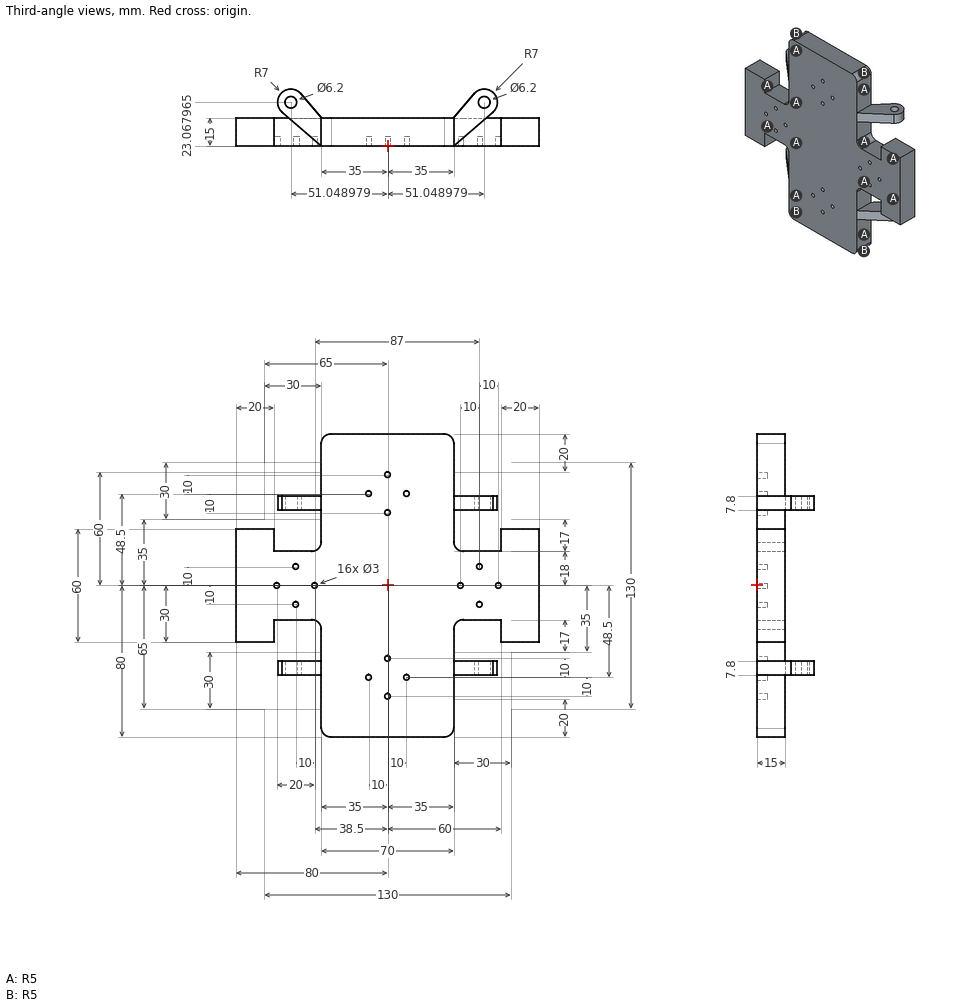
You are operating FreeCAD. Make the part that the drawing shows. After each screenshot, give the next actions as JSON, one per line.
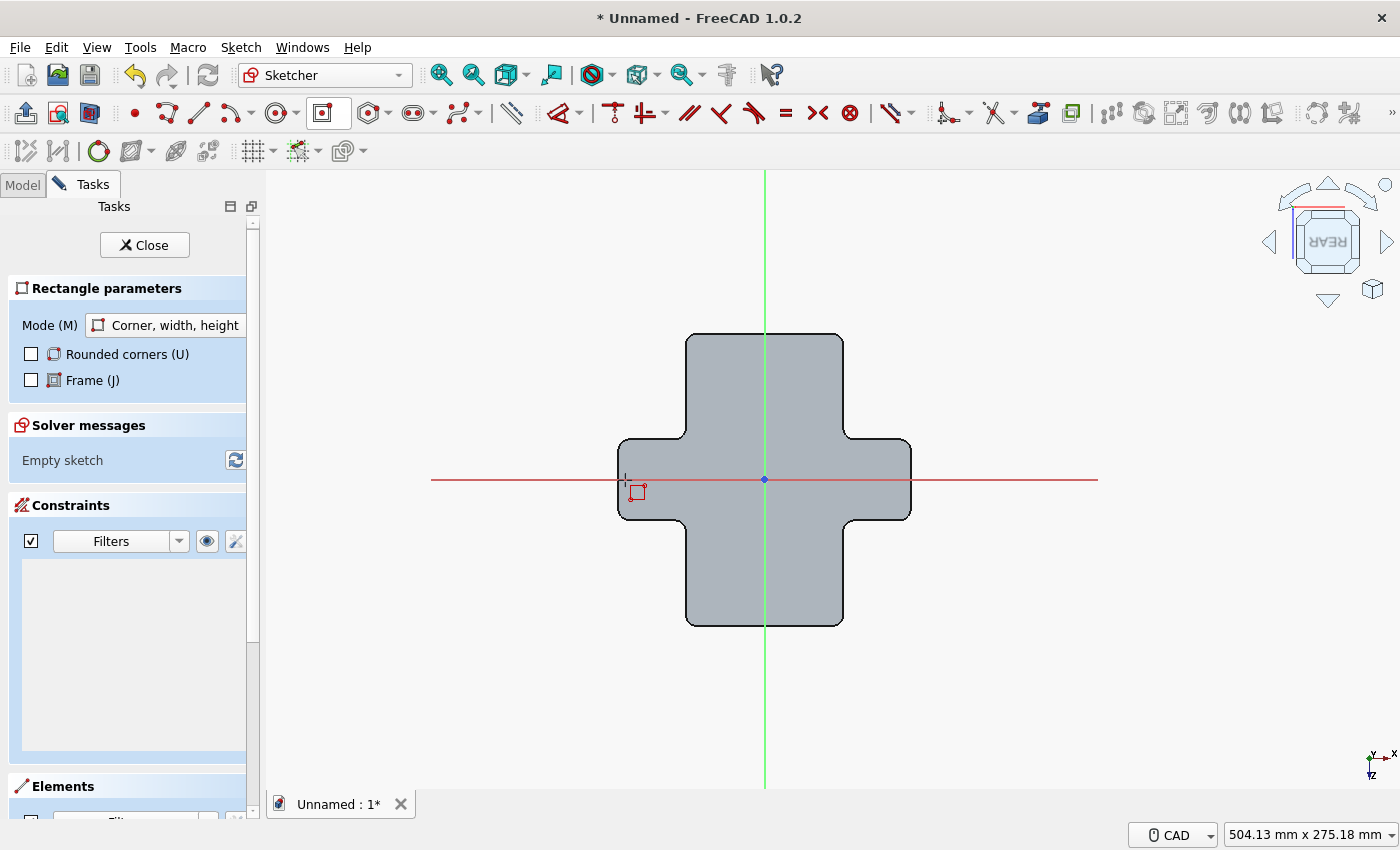
{"action": "left_click", "coordinate": [686, 300]}
{"action": "mouse_move", "coordinate": [843, 345]}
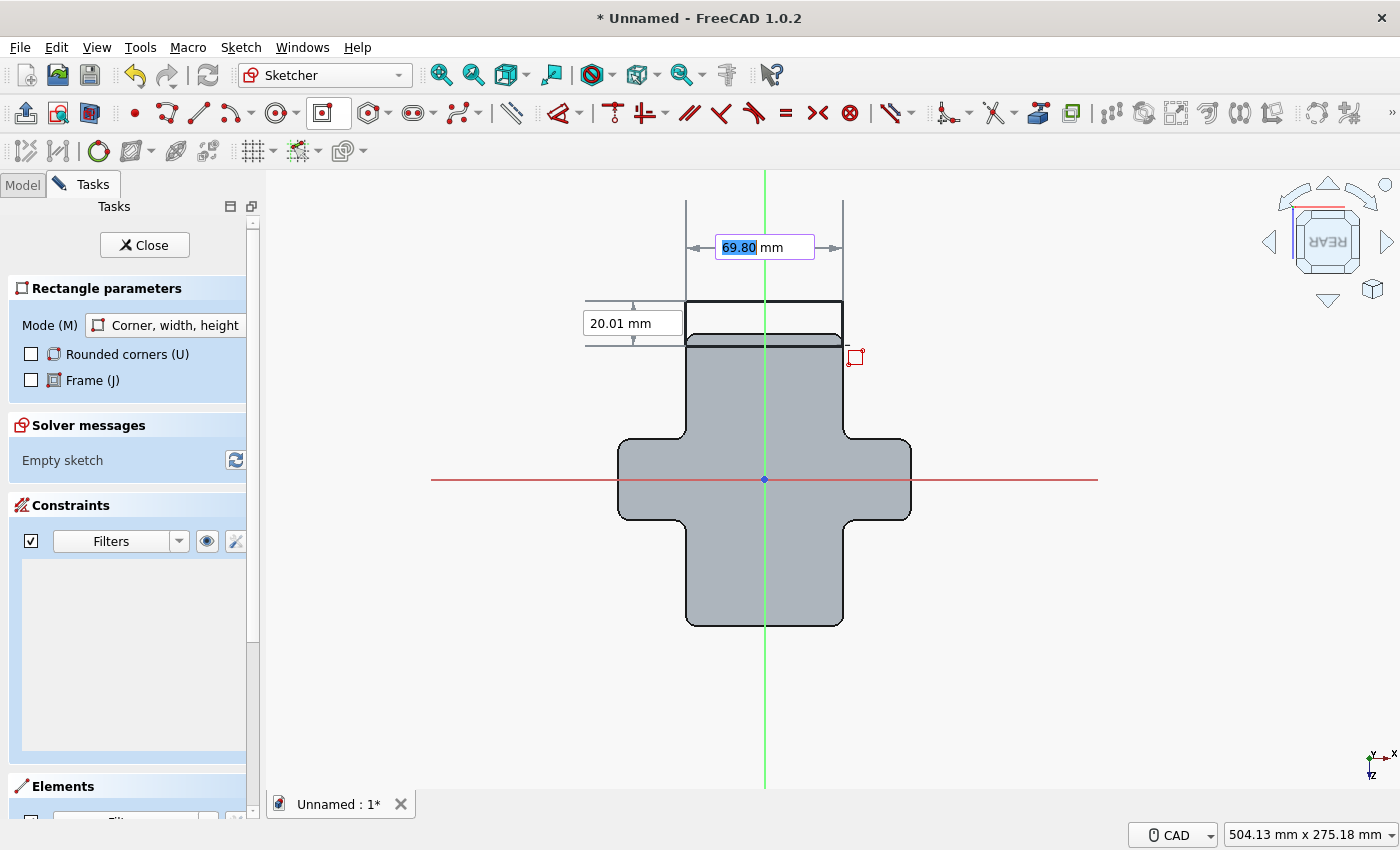
{"action": "type", "text": "70"}
{"action": "key", "text": "Tab"}
{"action": "type", "text": "20"}
{"action": "key", "text": "Return"}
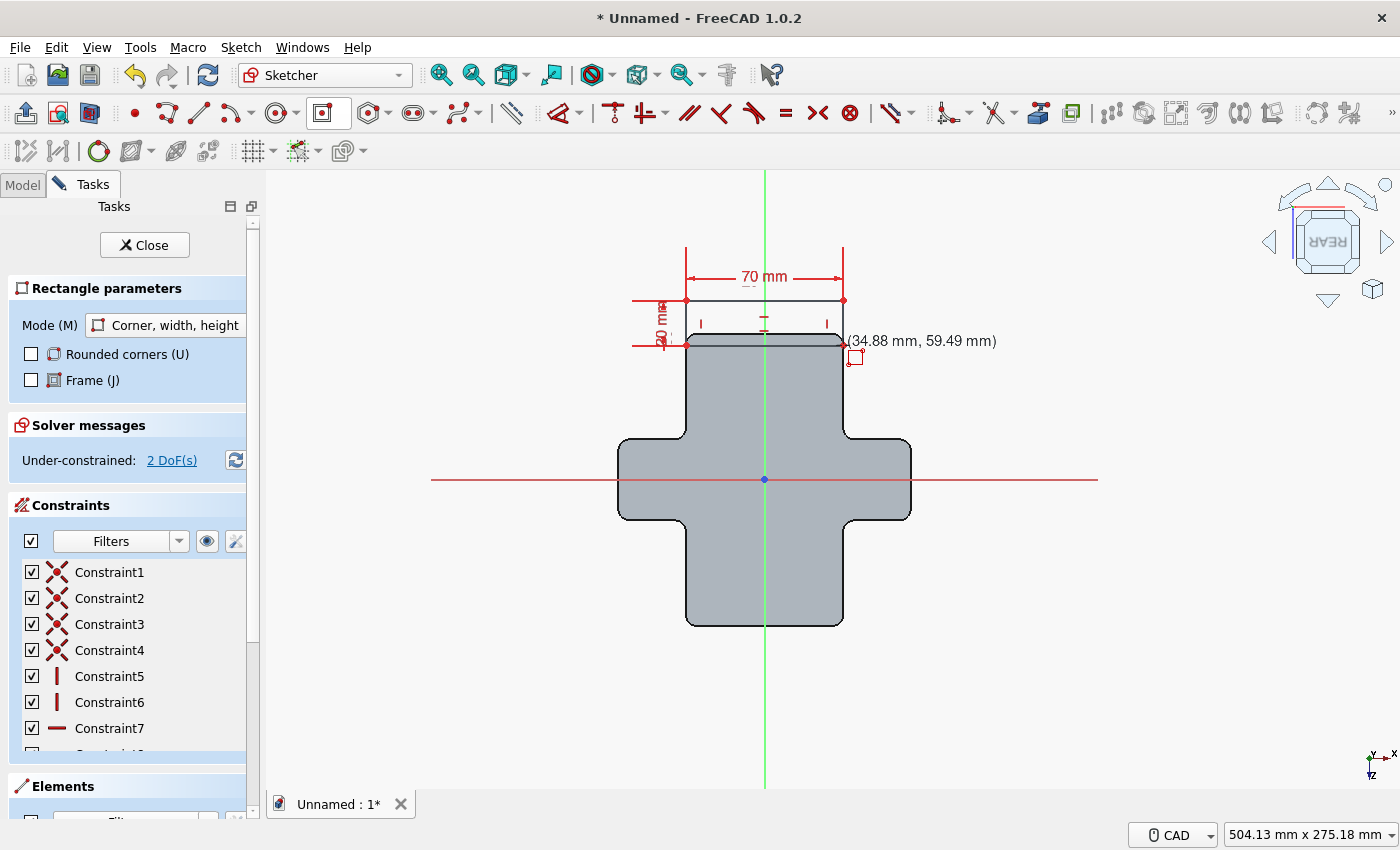
{"action": "left_click", "coordinate": [686, 615]}
{"action": "mouse_move", "coordinate": [843, 660]}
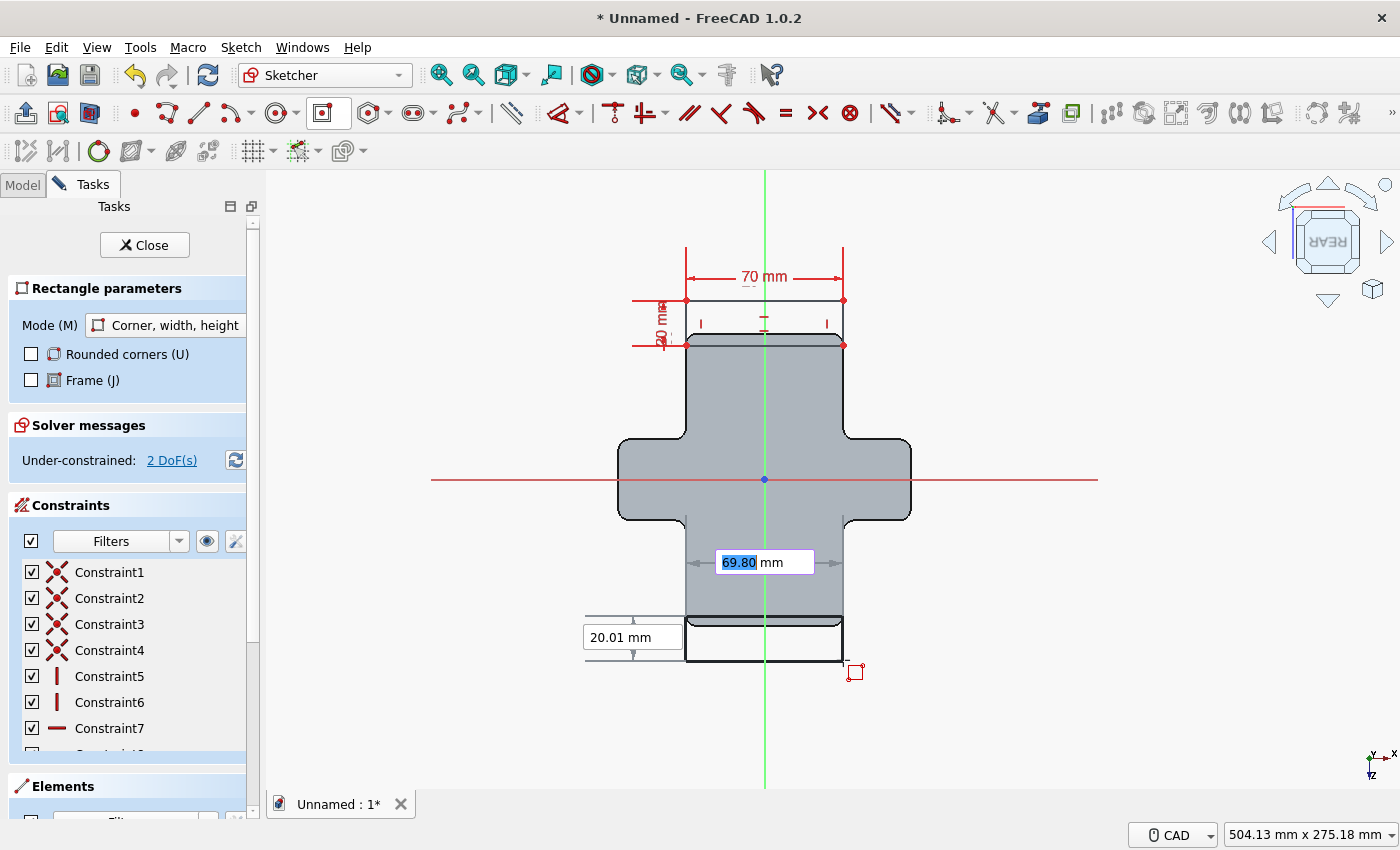
{"action": "type", "text": "70"}
{"action": "key", "text": "Tab"}
{"action": "type", "text": "20"}
{"action": "key", "text": "Return"}
{"action": "key", "text": "Escape"}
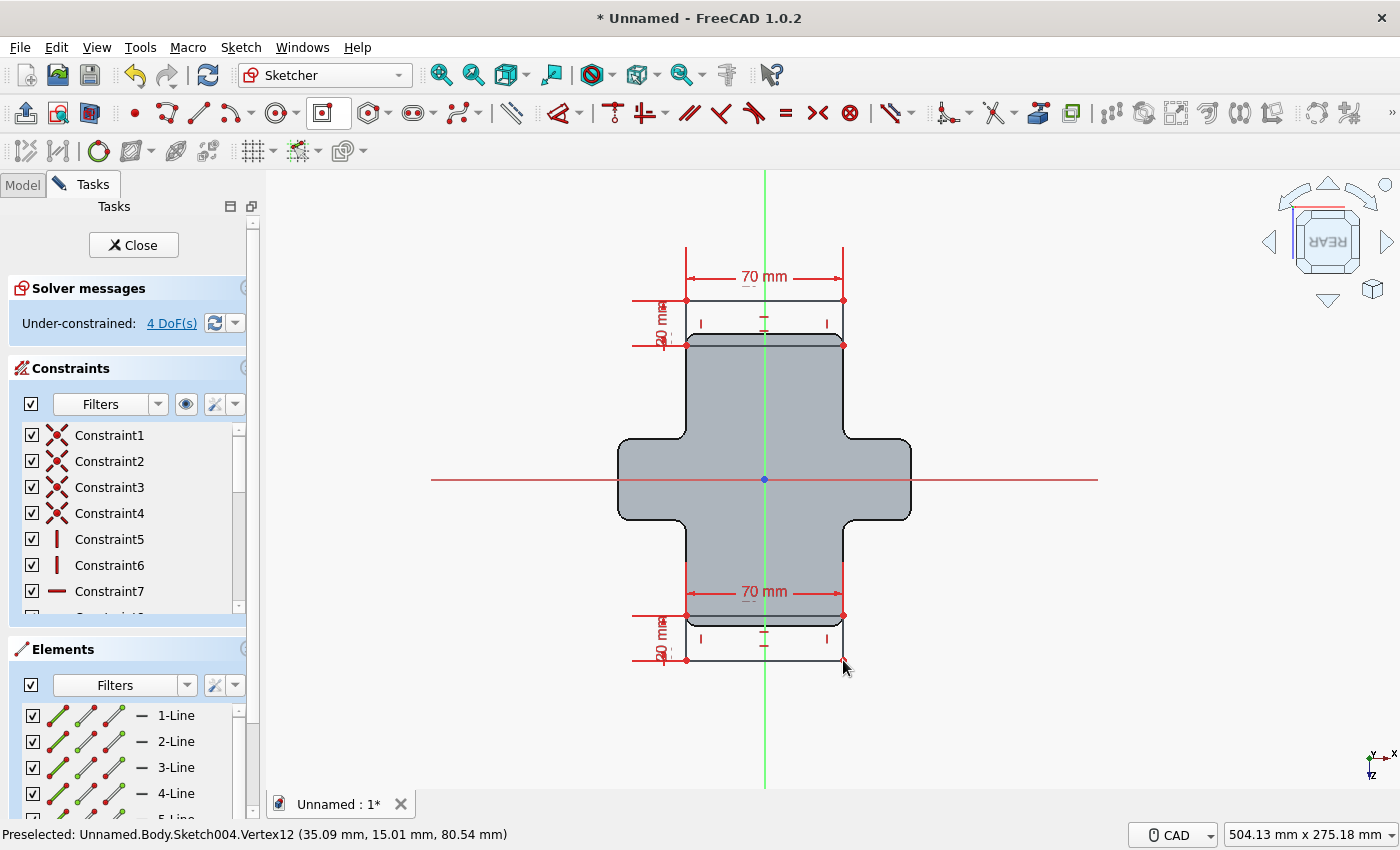
{"action": "key", "text": "d"}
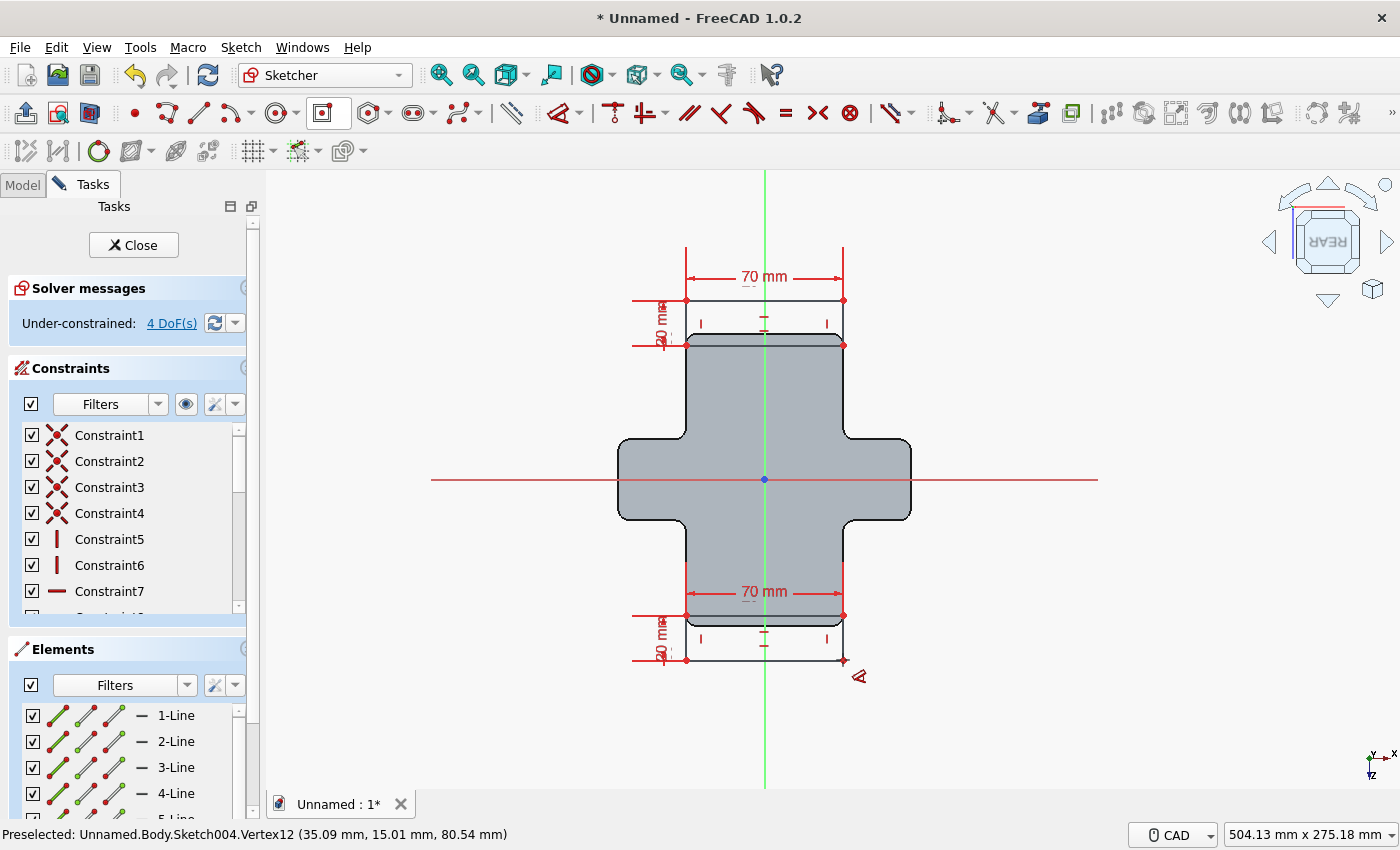
{"action": "left_click", "coordinate": [686, 301]}
{"action": "left_click", "coordinate": [725, 267]}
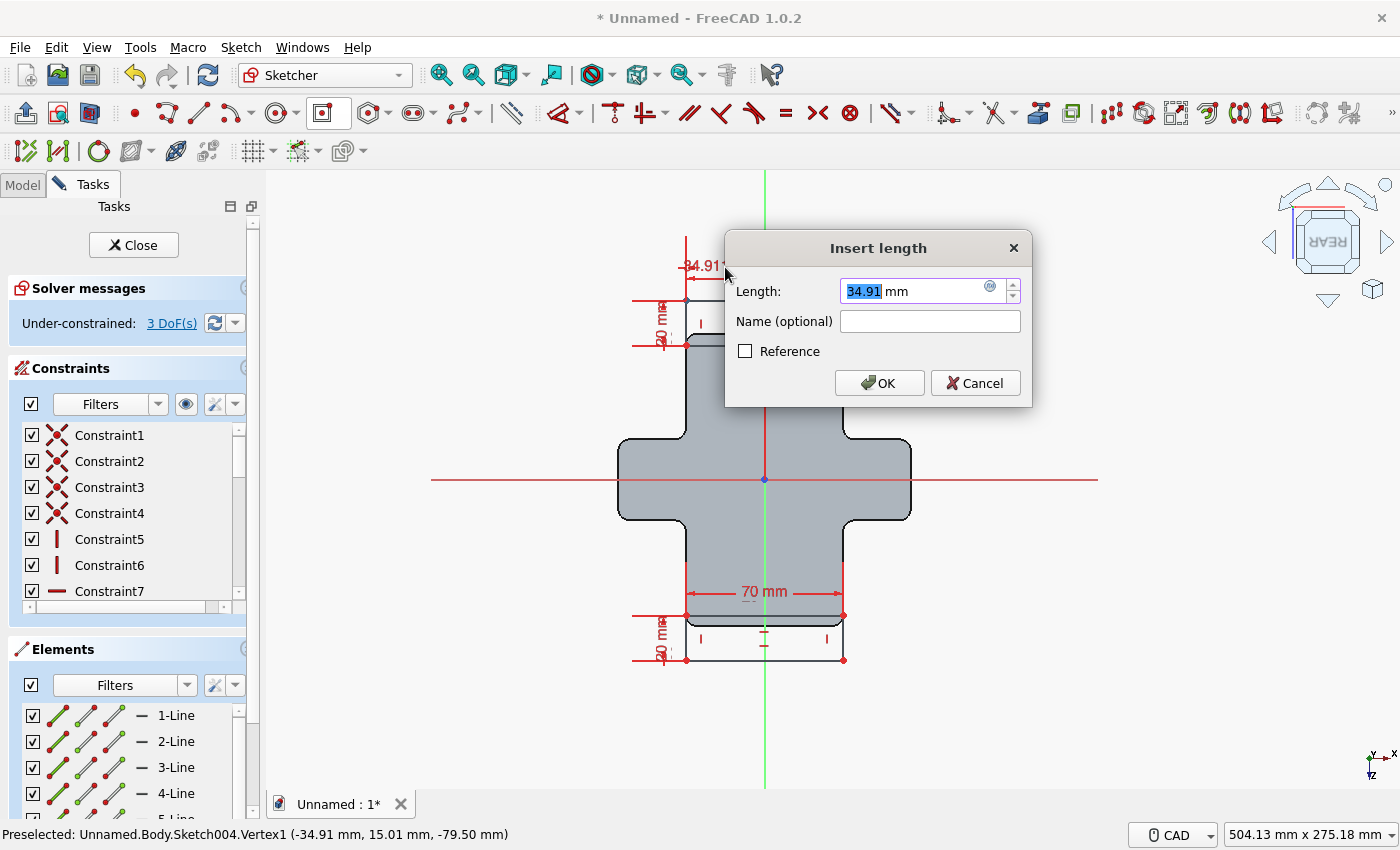
{"action": "type", "text": "35"}
{"action": "key", "text": "Return"}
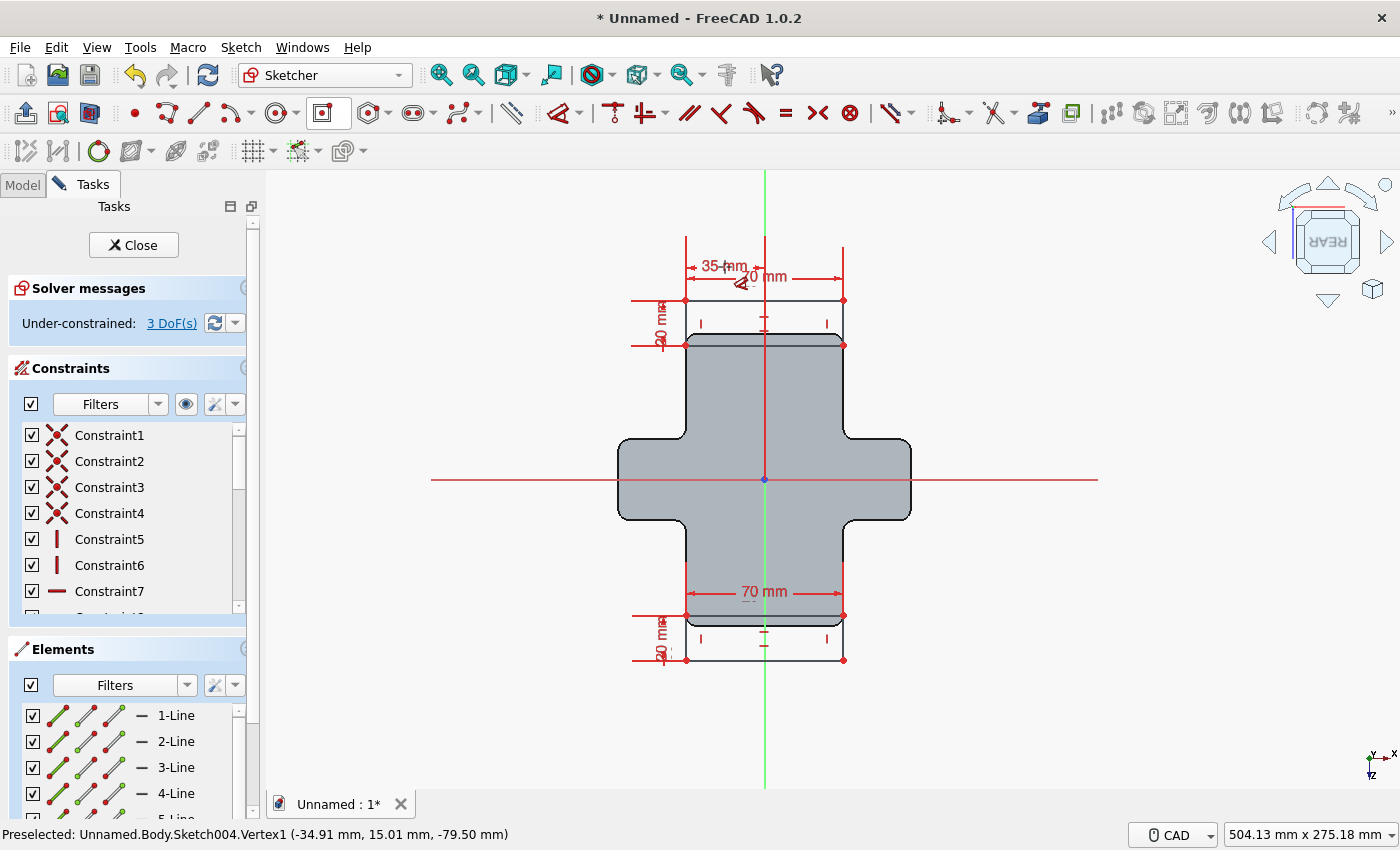
{"action": "left_click", "coordinate": [686, 301]}
{"action": "left_click", "coordinate": [652, 390]}